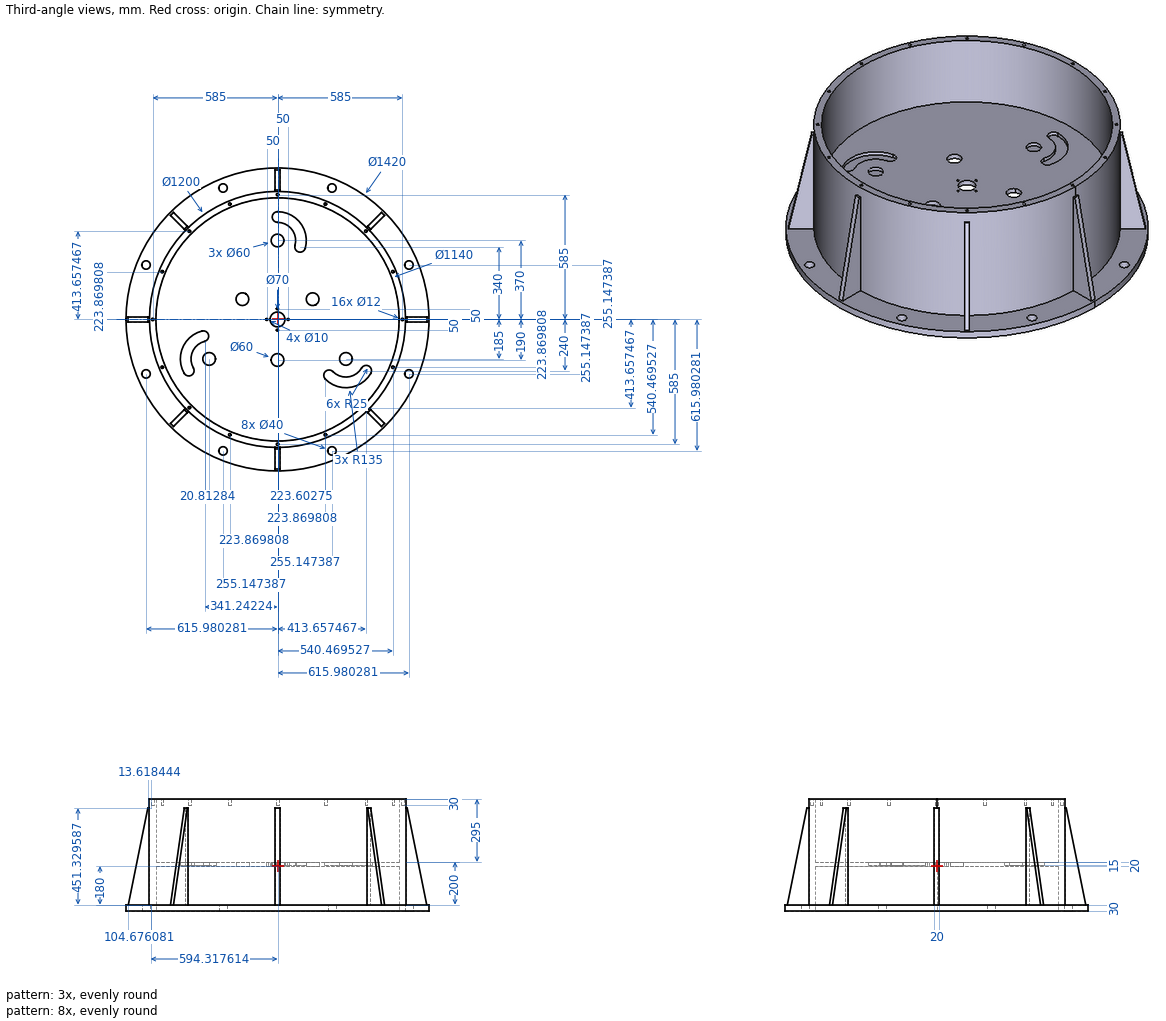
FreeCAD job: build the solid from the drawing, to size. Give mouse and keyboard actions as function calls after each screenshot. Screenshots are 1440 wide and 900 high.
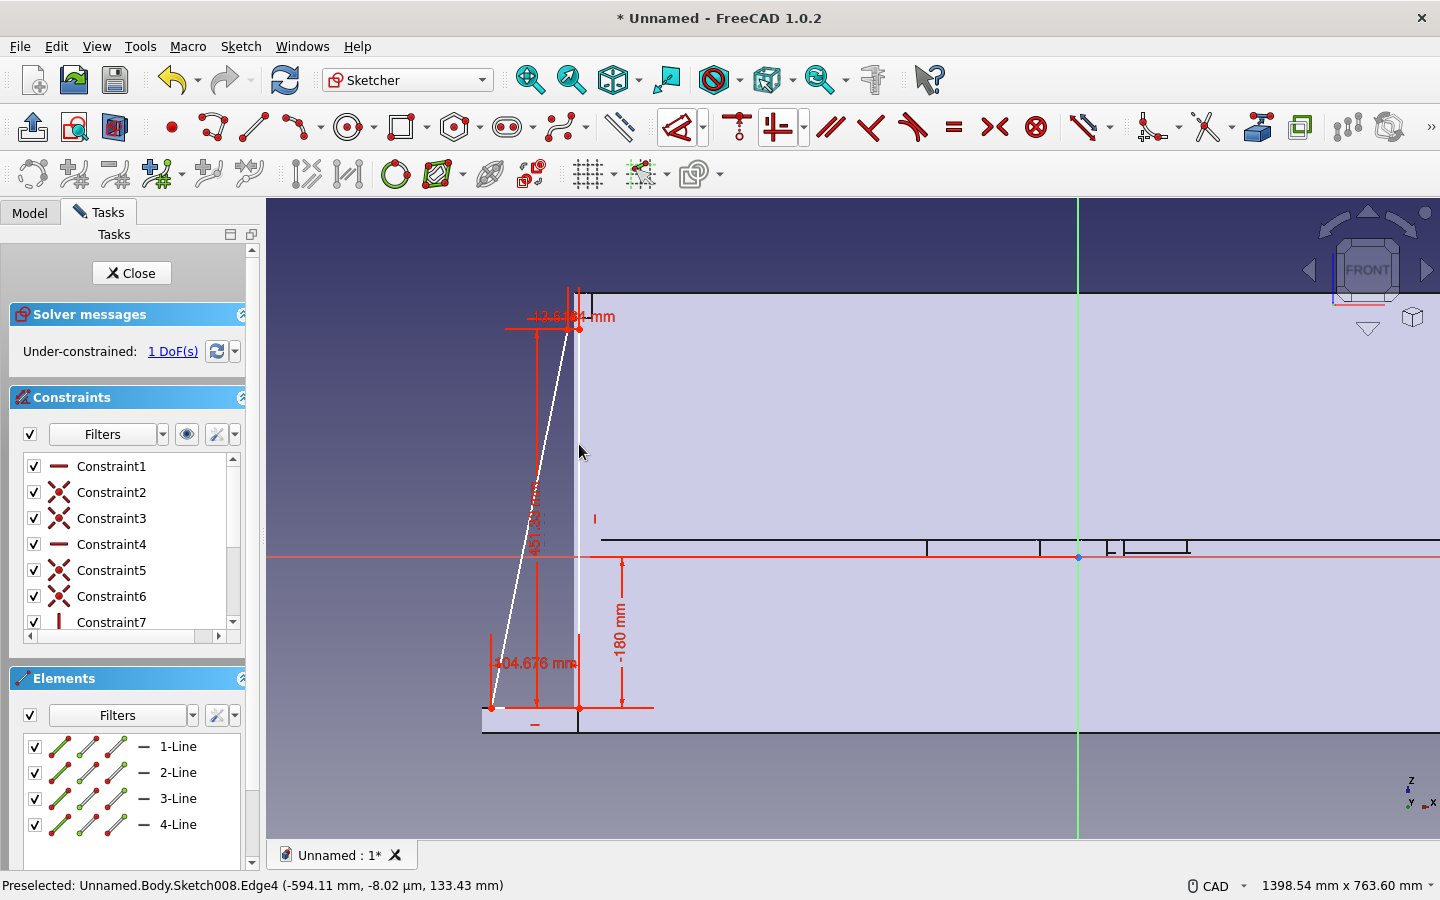
click(579, 708)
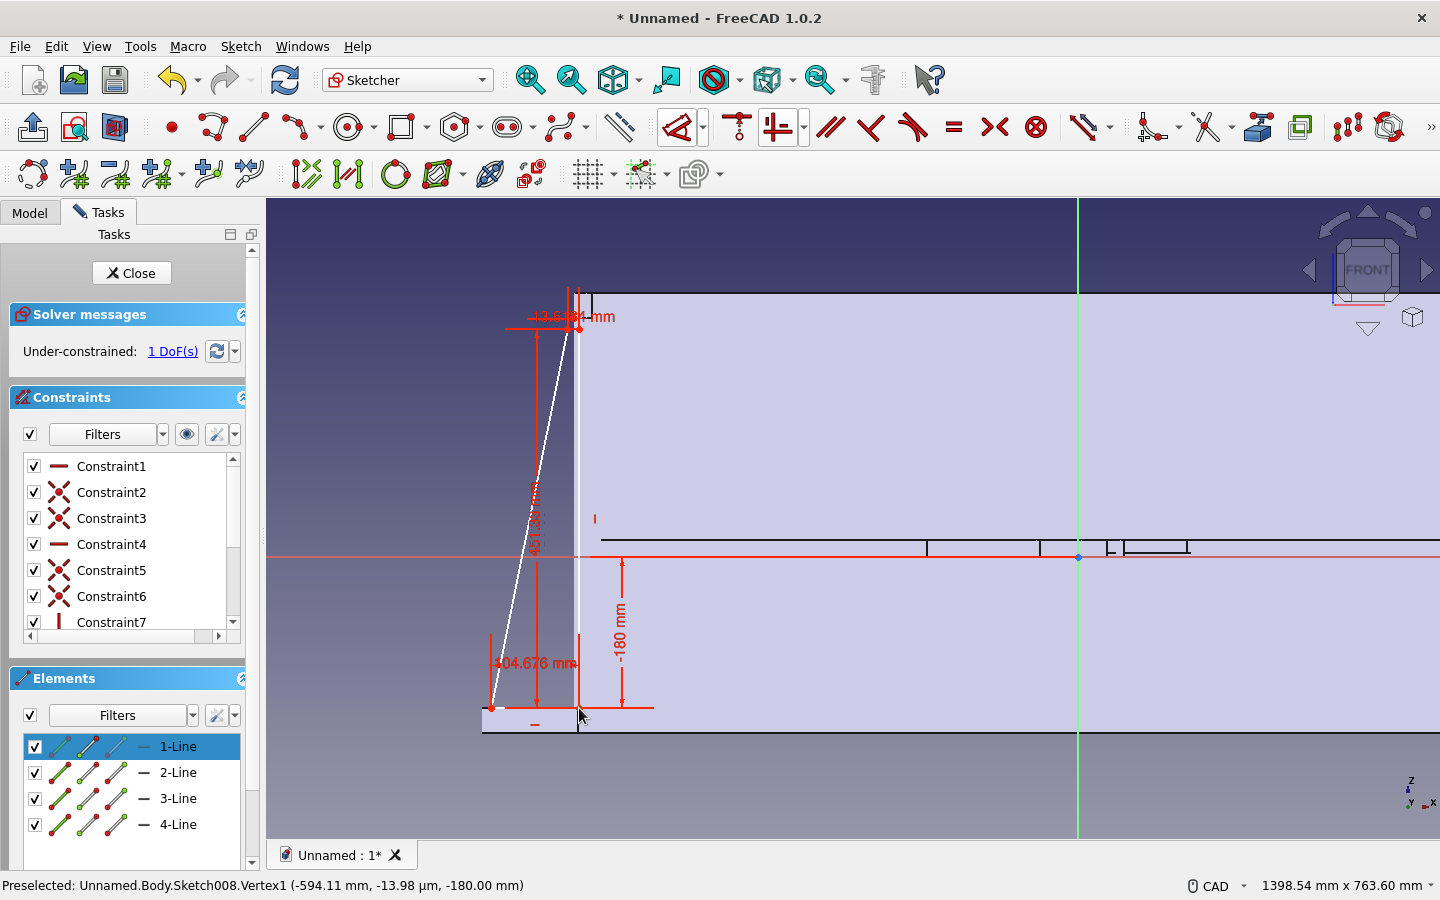
click(702, 128)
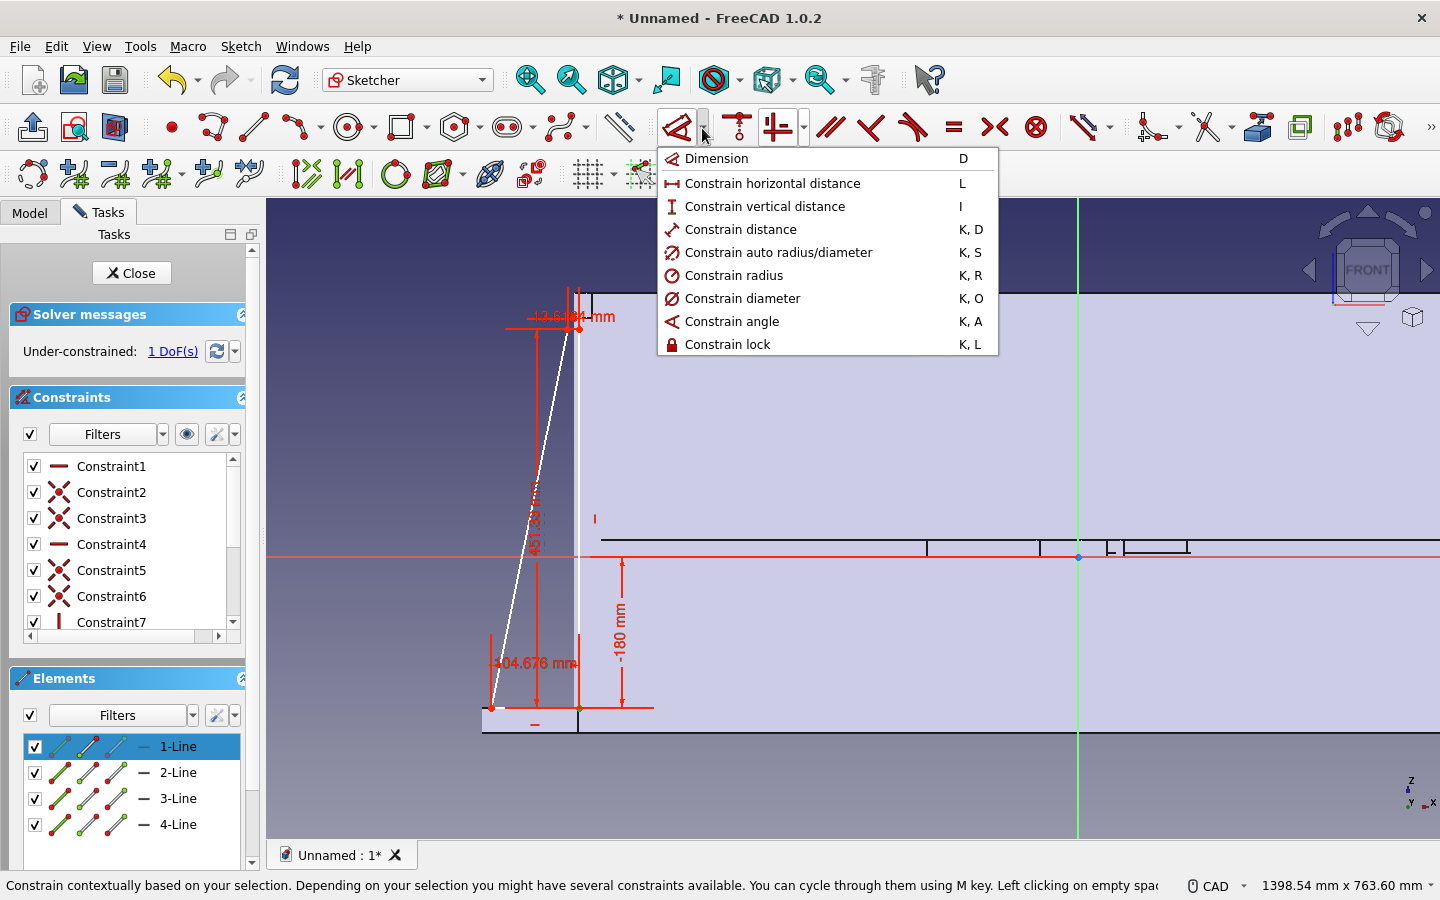
click(828, 184)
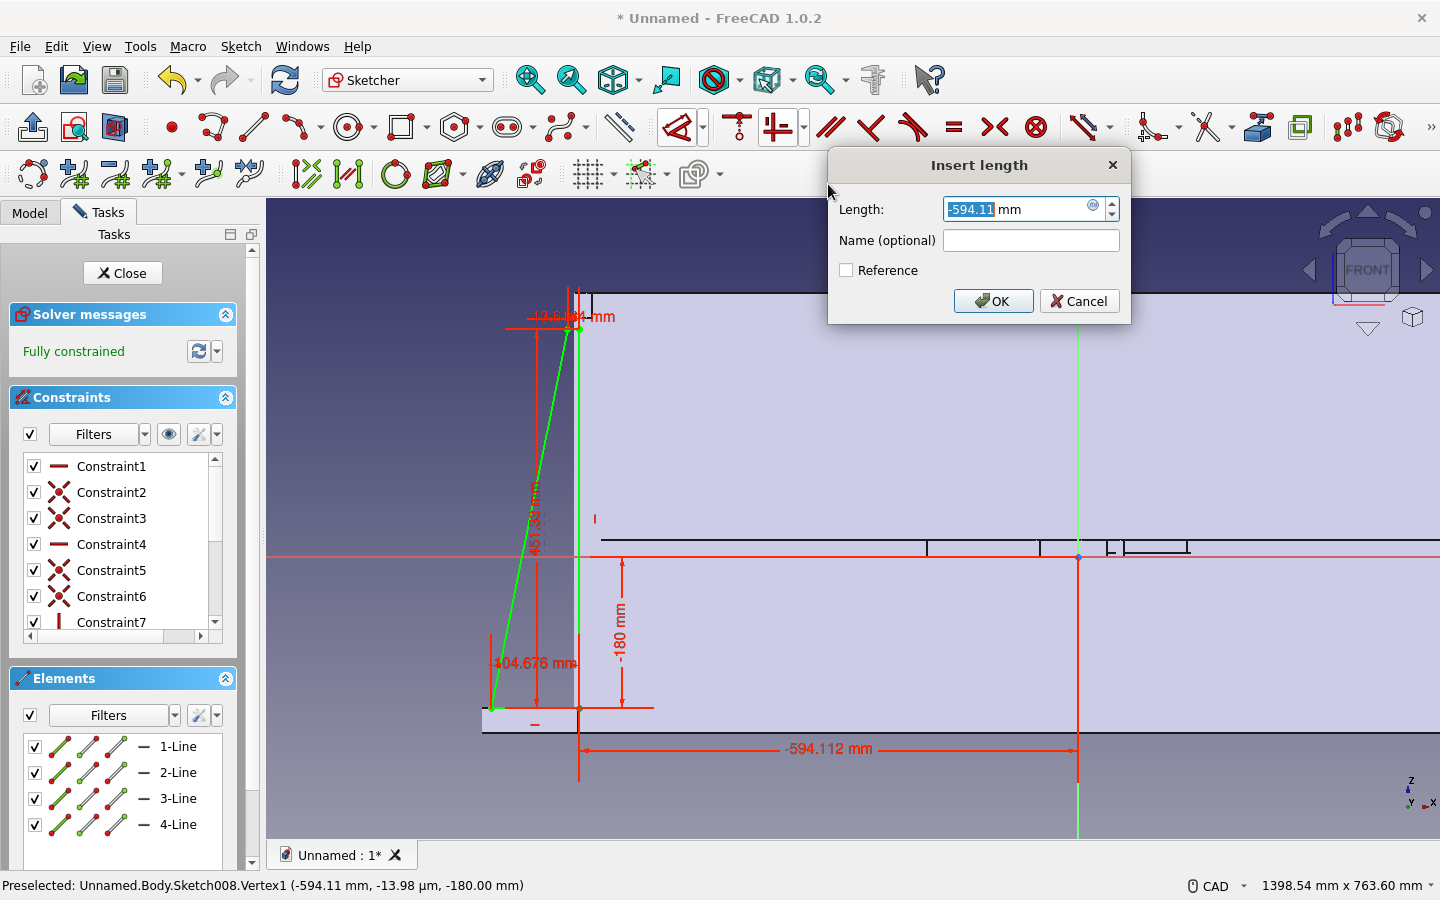
text(-594.317614)
key(Return)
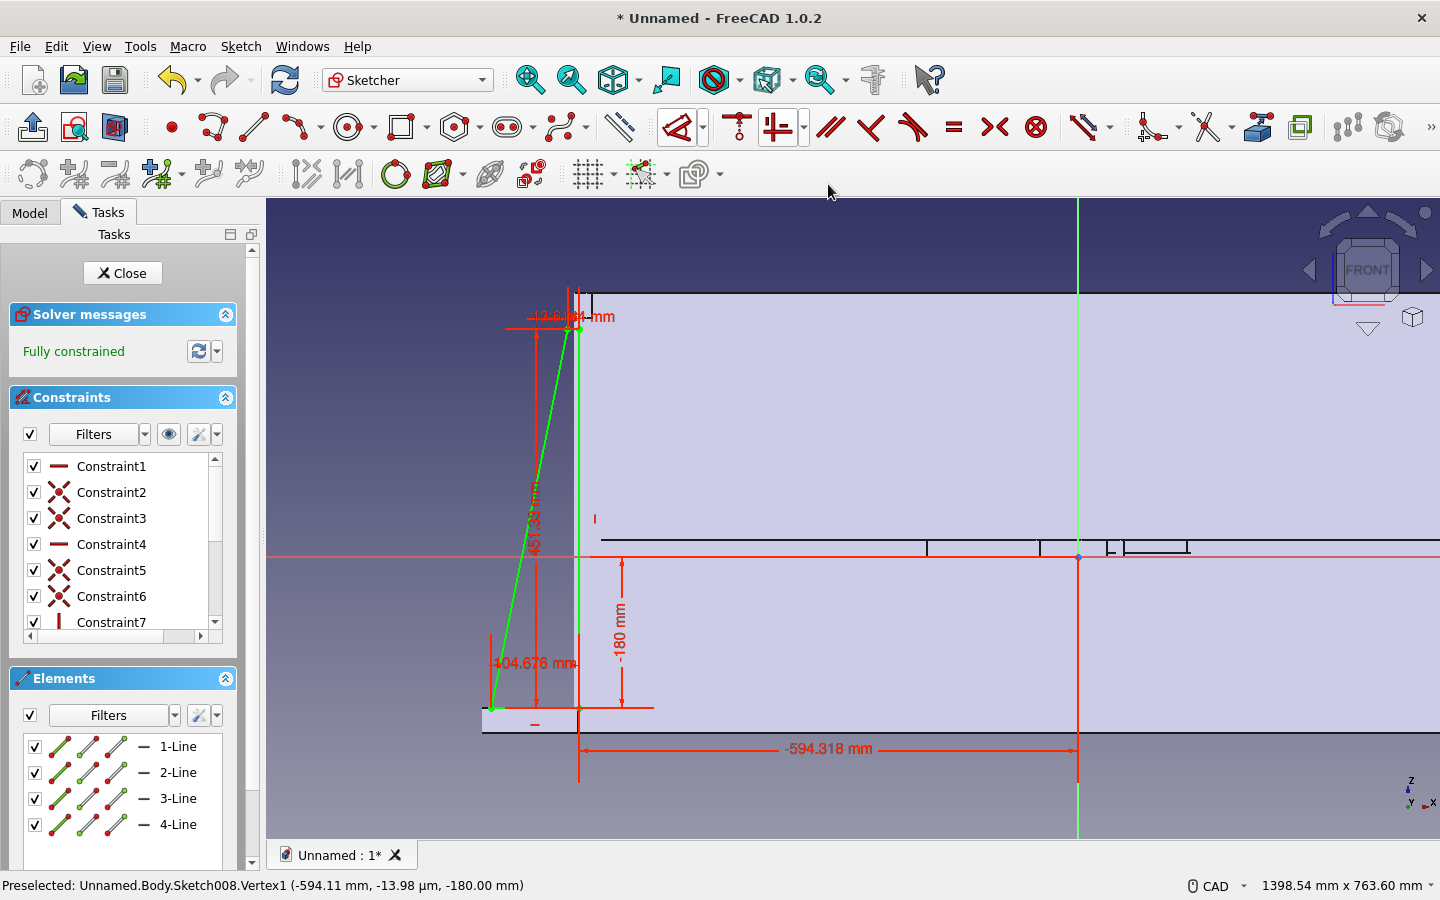
click(123, 273)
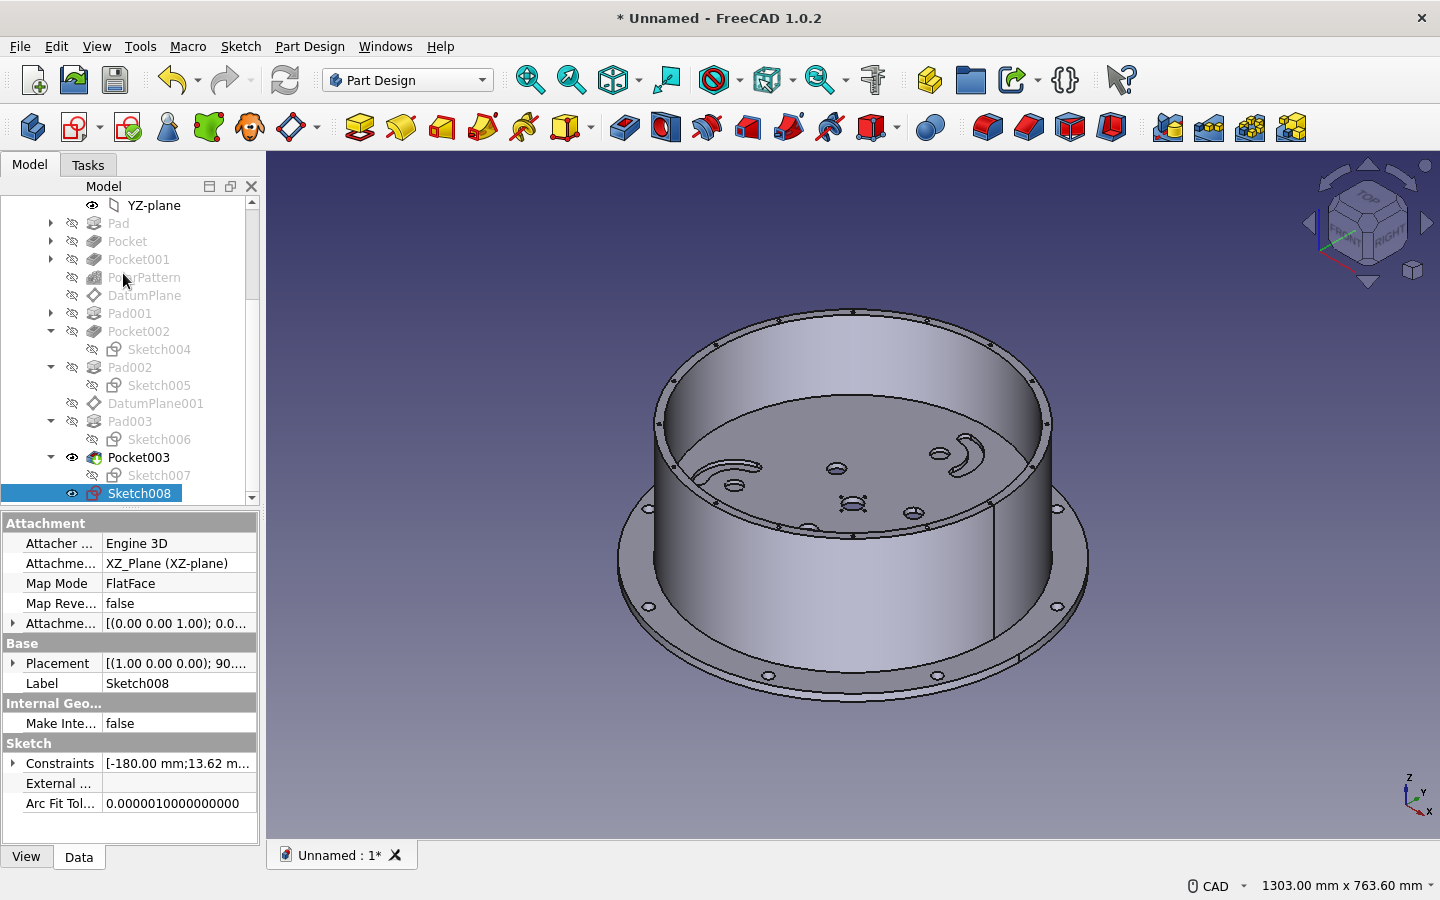
click(360, 128)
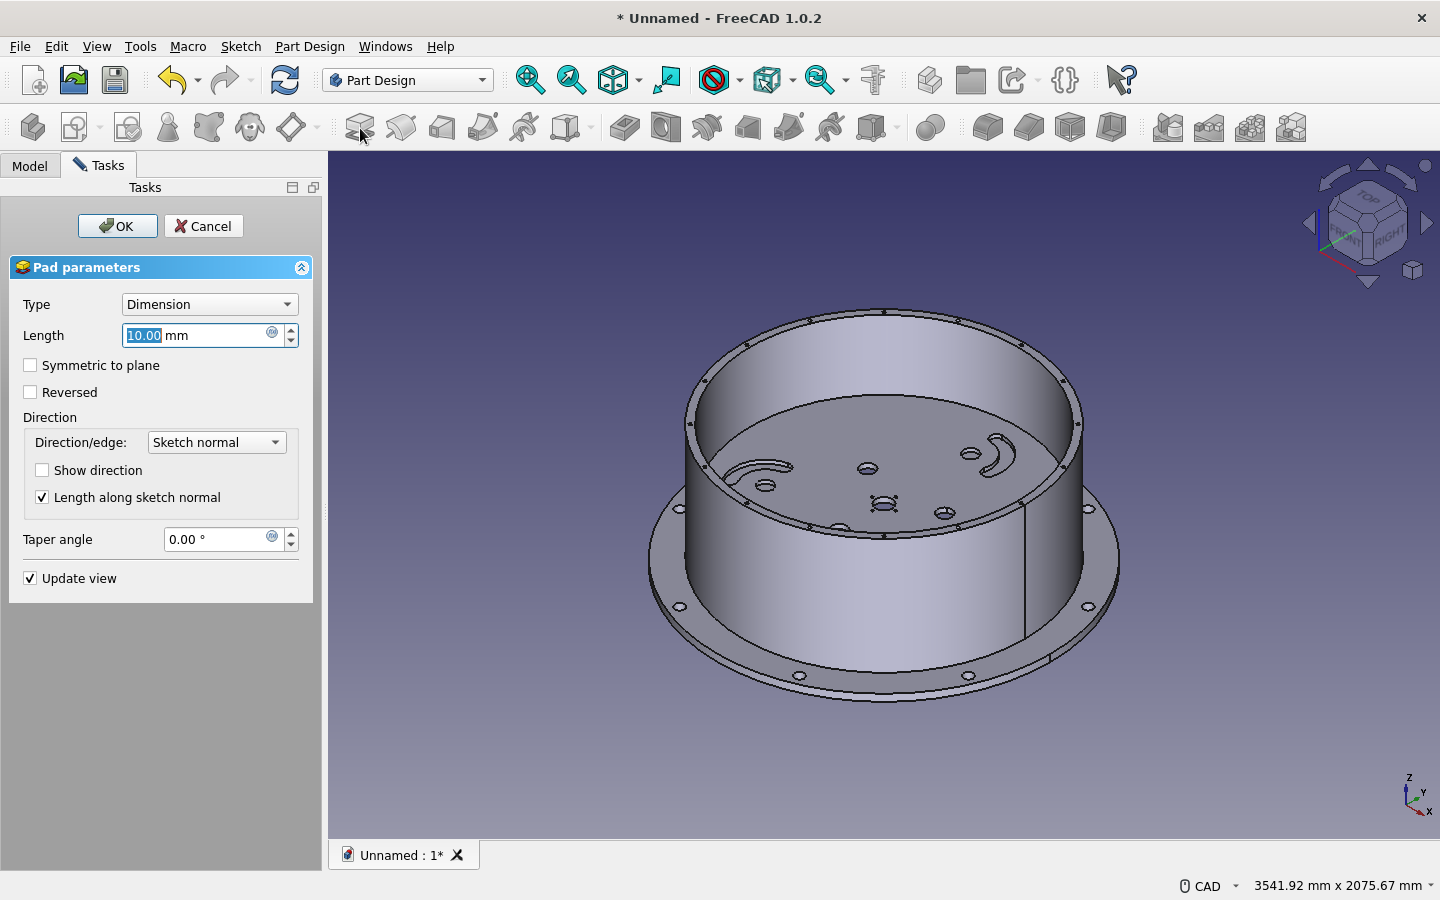
text(20)
key(Tab)